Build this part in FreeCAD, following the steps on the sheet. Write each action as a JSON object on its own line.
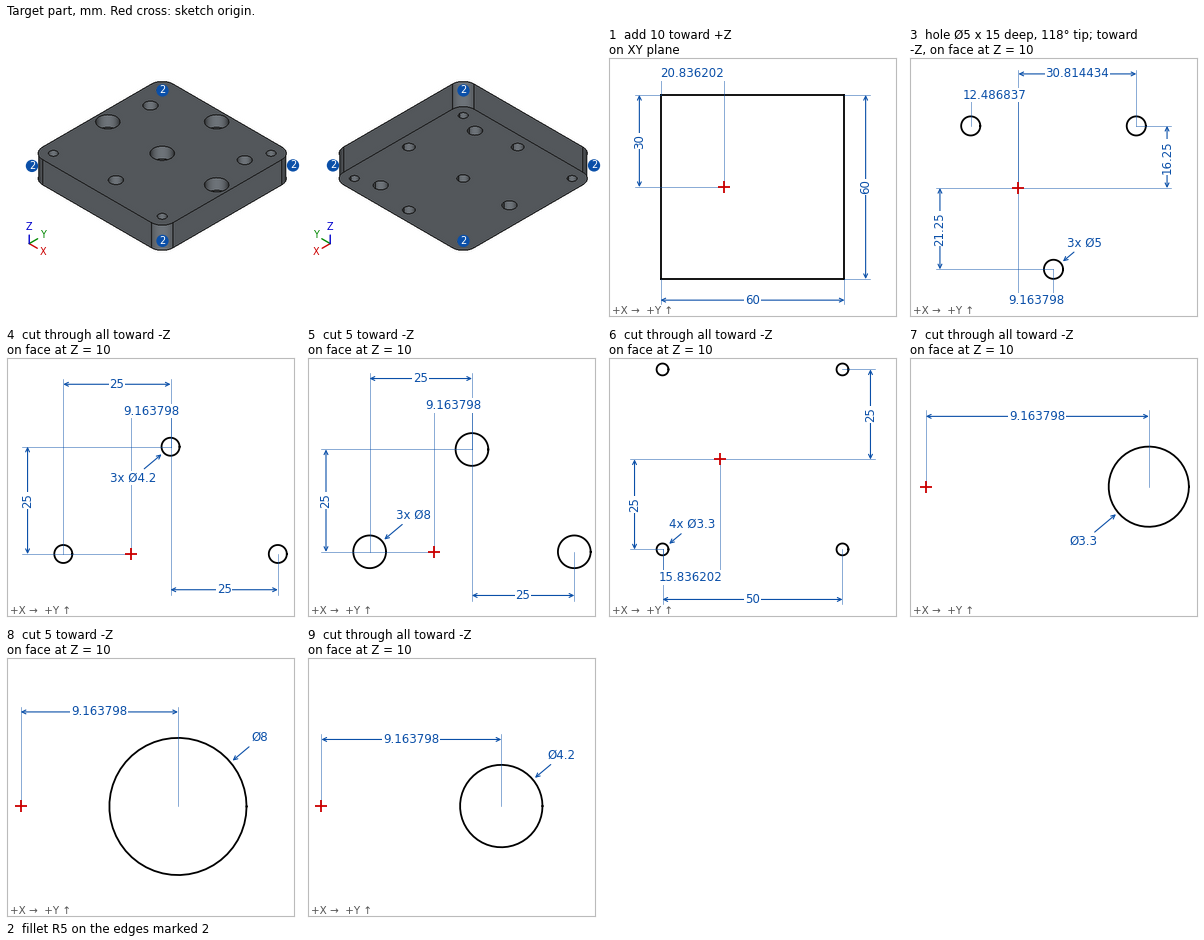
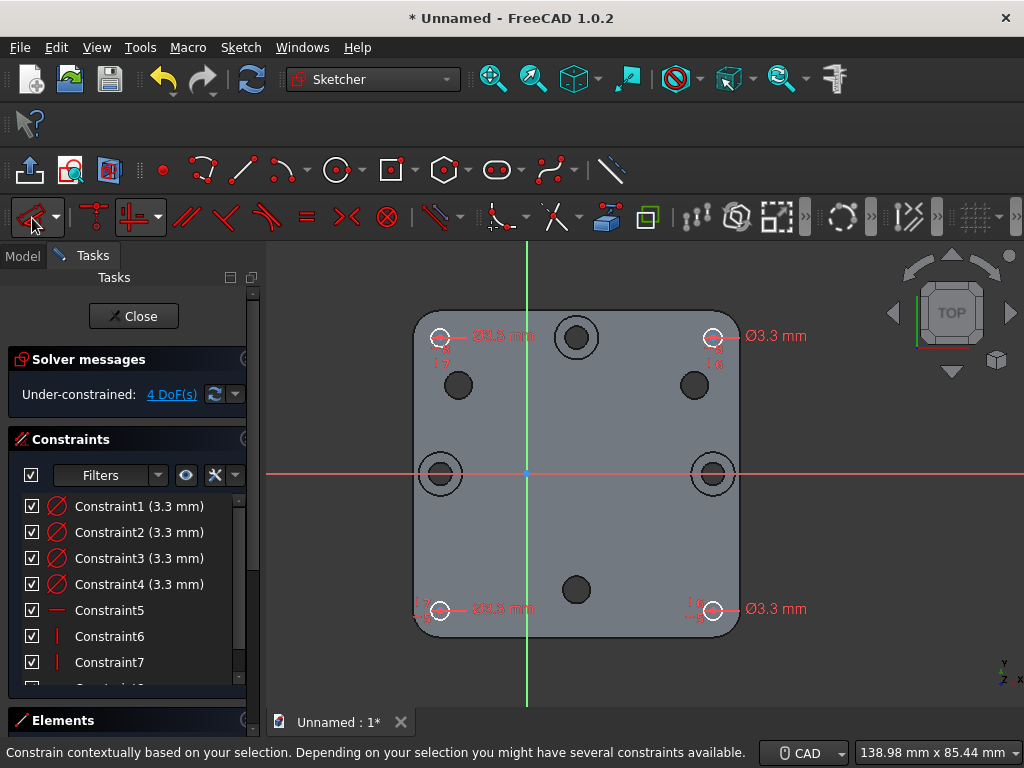
{"action": "left_click", "coordinate": [440, 611]}
{"action": "left_click", "coordinate": [406, 542]}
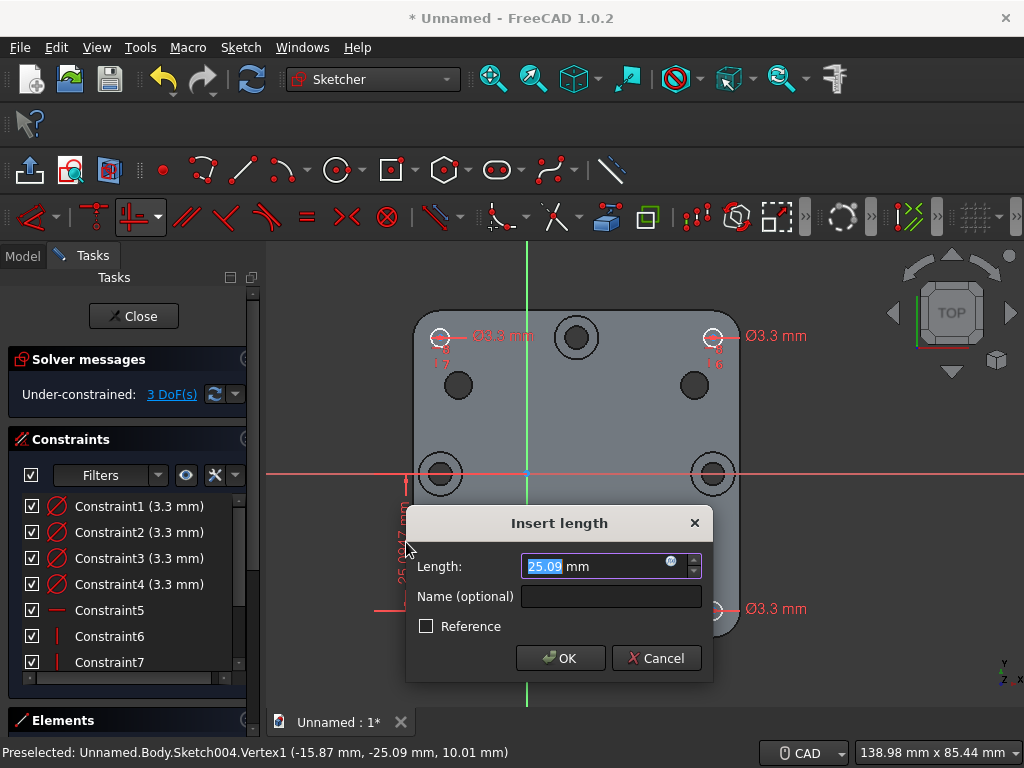
{"action": "type", "text": "25"}
{"action": "key", "text": "Return"}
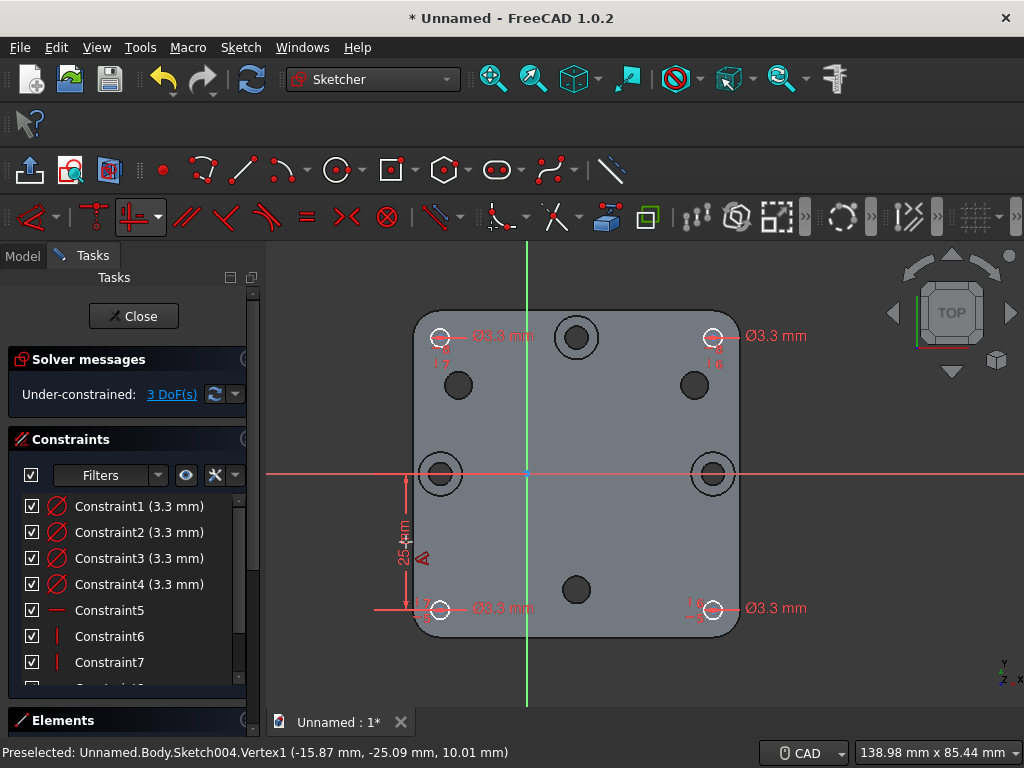
{"action": "left_click", "coordinate": [713, 338]}
{"action": "left_click", "coordinate": [747, 406]}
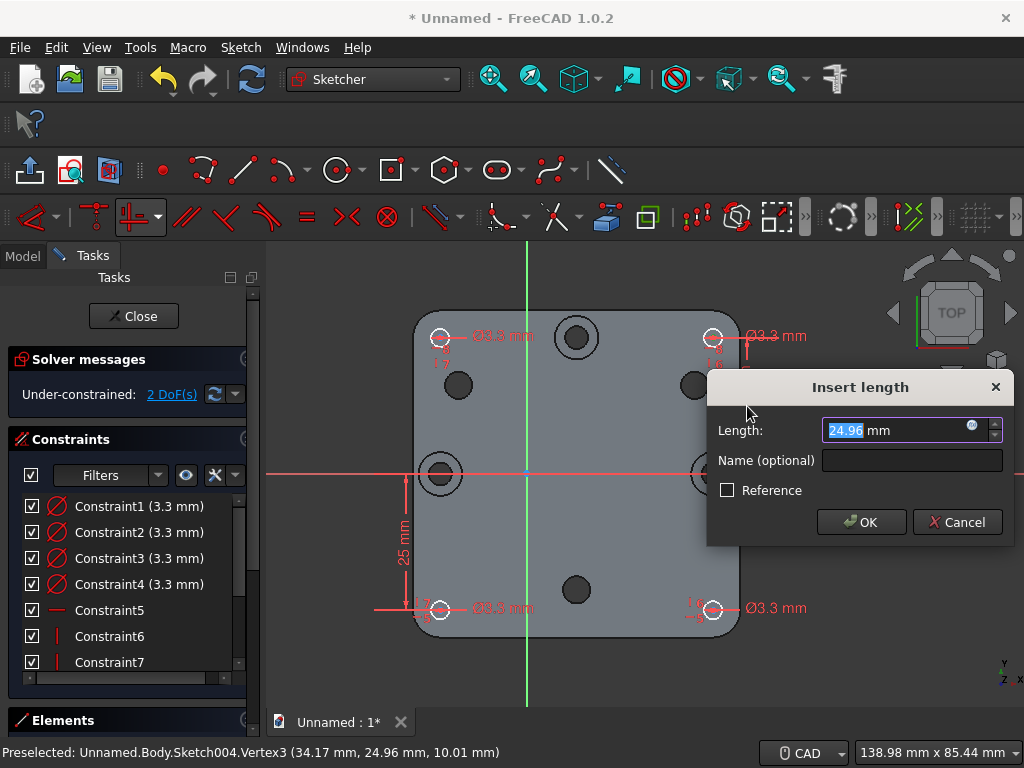
{"action": "type", "text": "25"}
{"action": "key", "text": "Return"}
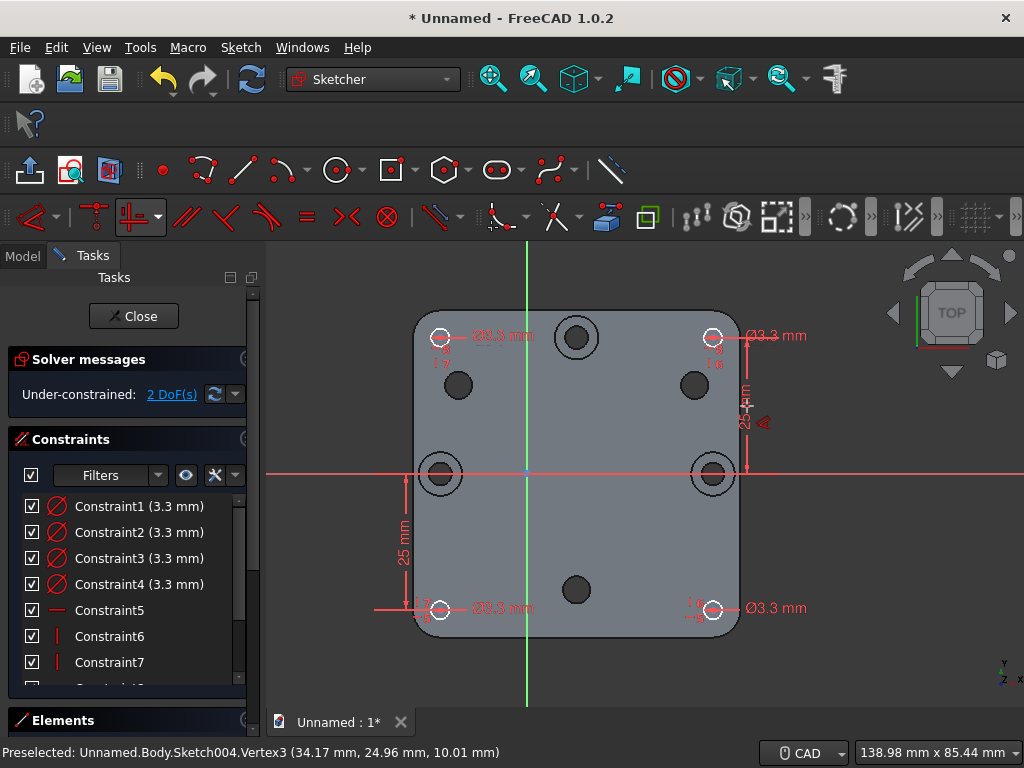
{"action": "left_click", "coordinate": [440, 610]}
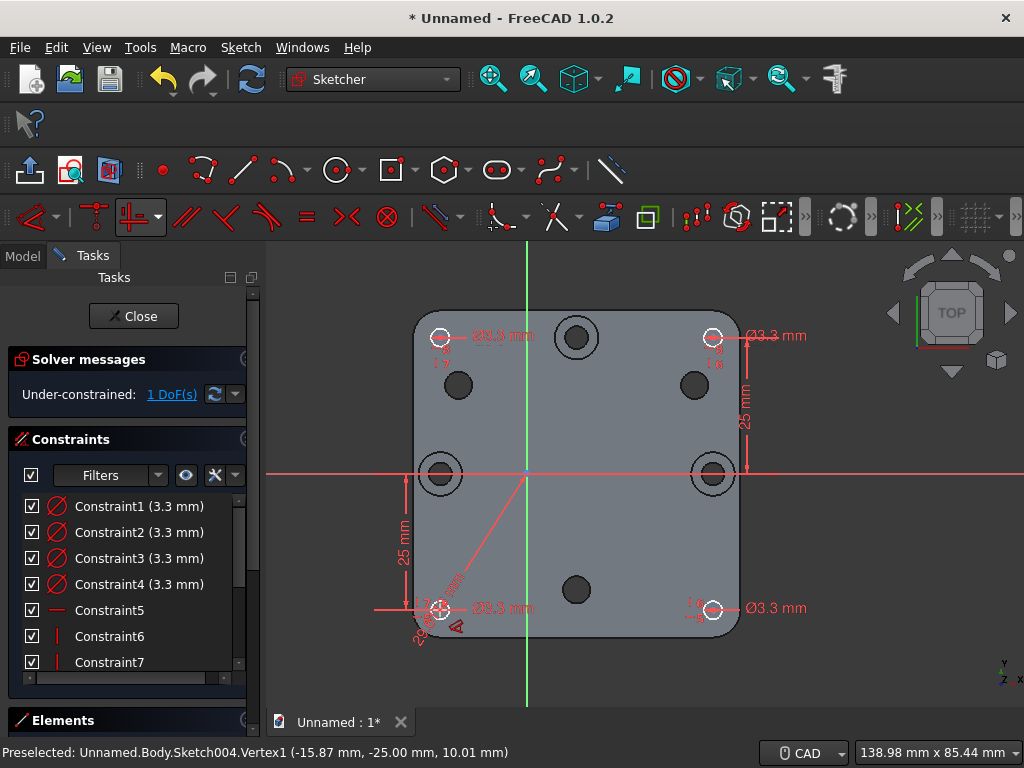
{"action": "left_click", "coordinate": [713, 610]}
{"action": "left_click", "coordinate": [577, 644]}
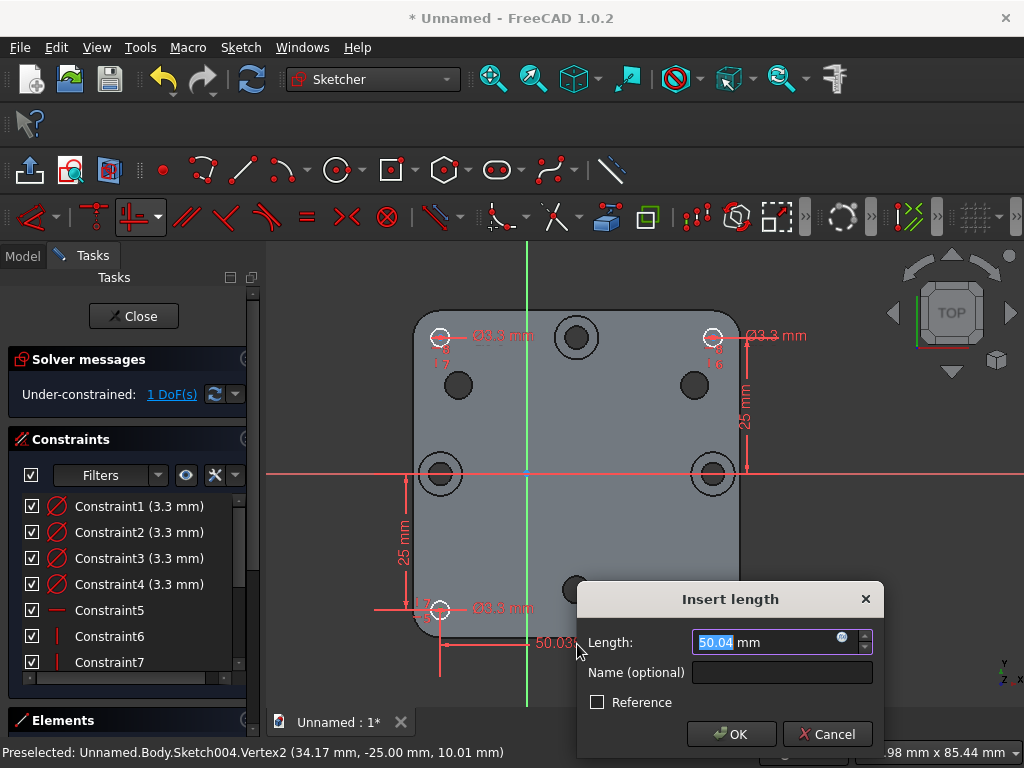
{"action": "type", "text": "50"}
{"action": "key", "text": "Return"}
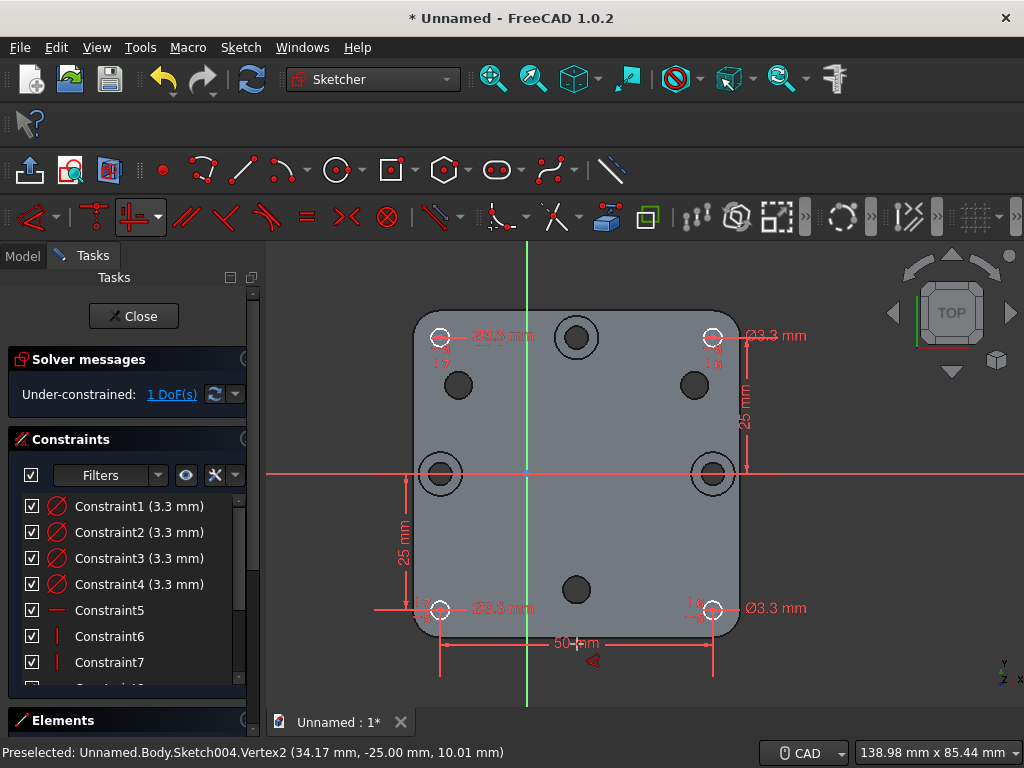
{"action": "left_click", "coordinate": [440, 610]}
{"action": "left_click", "coordinate": [483, 644]}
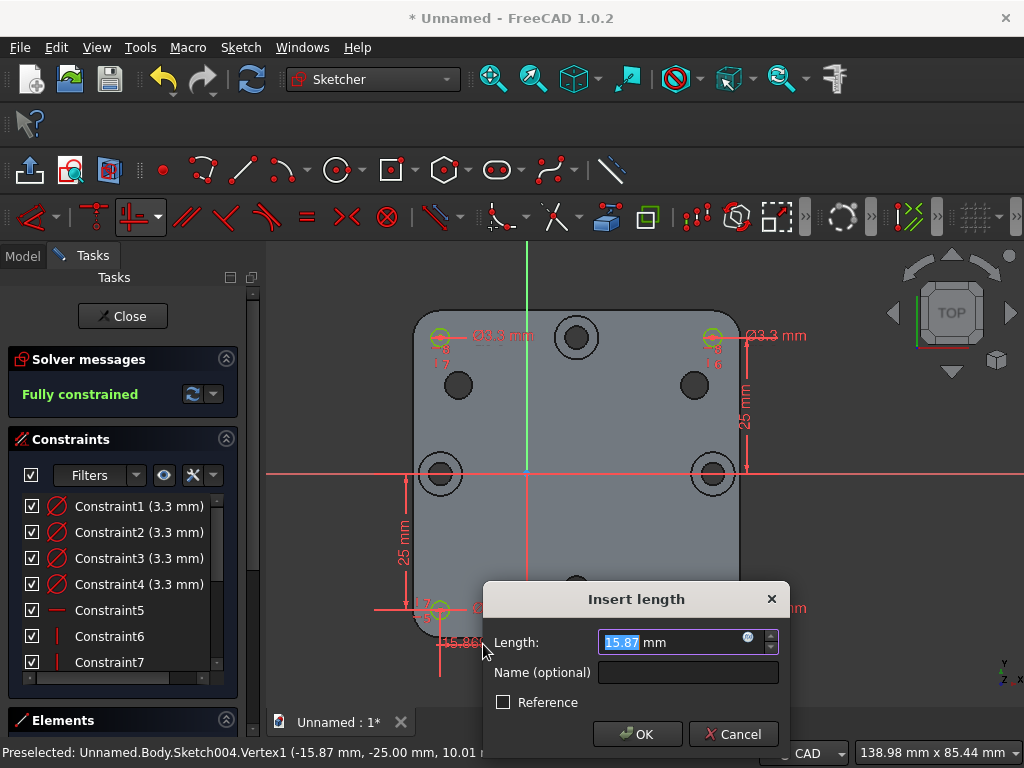
{"action": "type", "text": "15.836202"}
{"action": "key", "text": "Return"}
{"action": "key", "text": "Escape"}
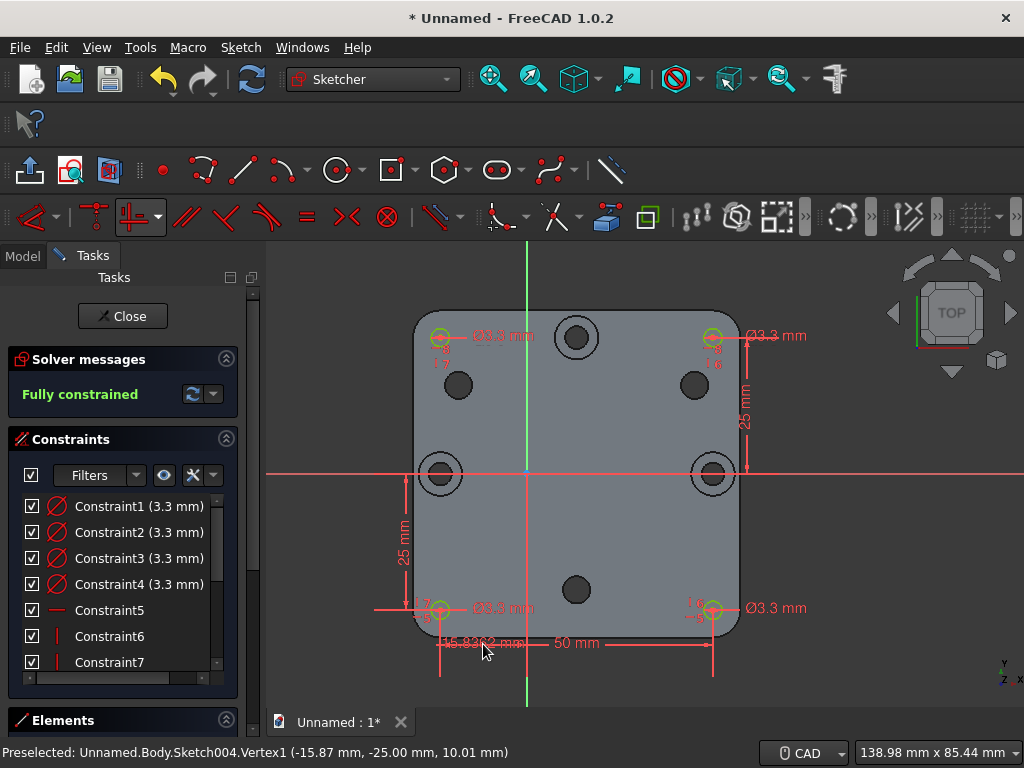
{"action": "left_click", "coordinate": [123, 316]}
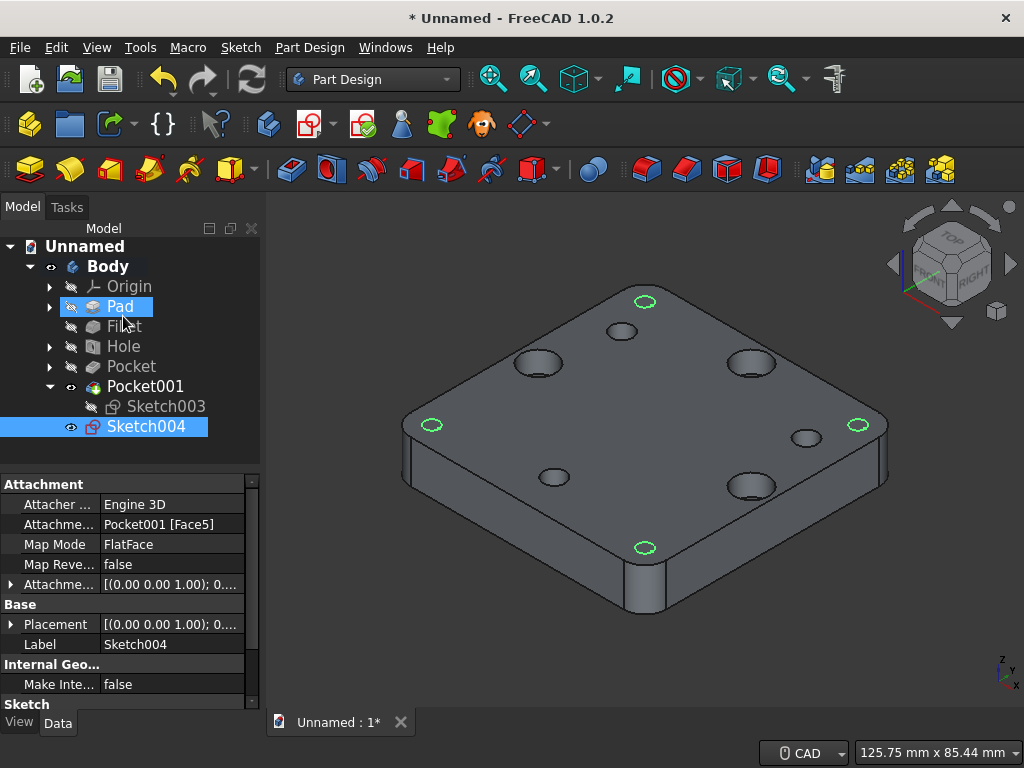
{"action": "left_click", "coordinate": [292, 170]}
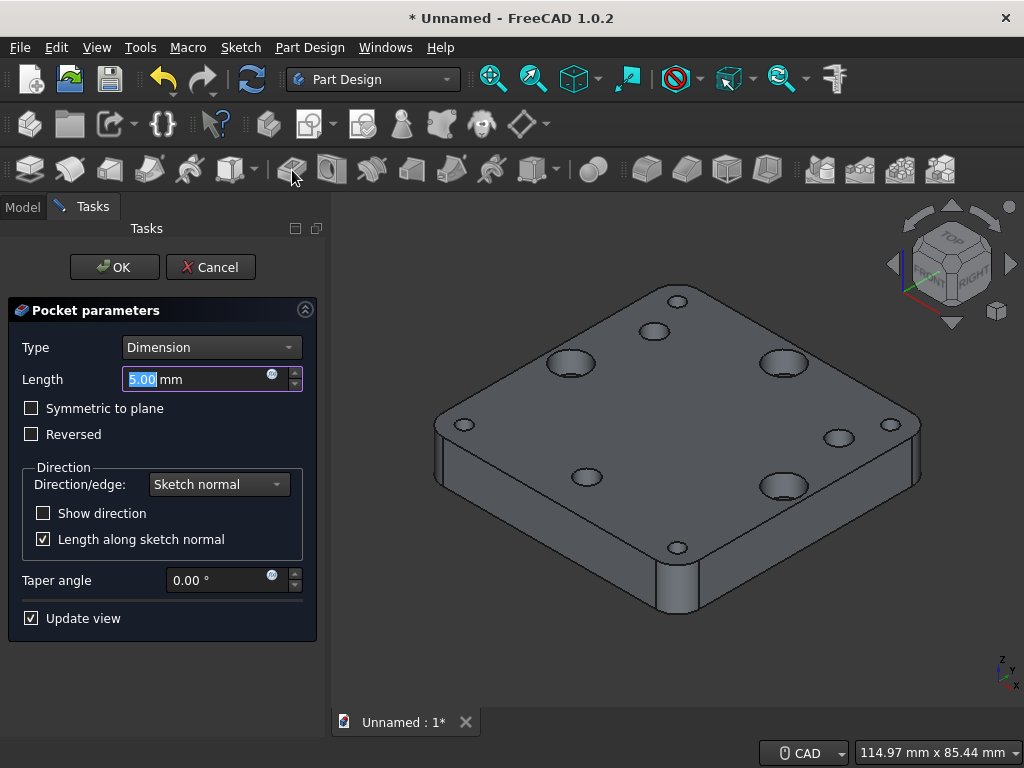
{"action": "left_click", "coordinate": [212, 348]}